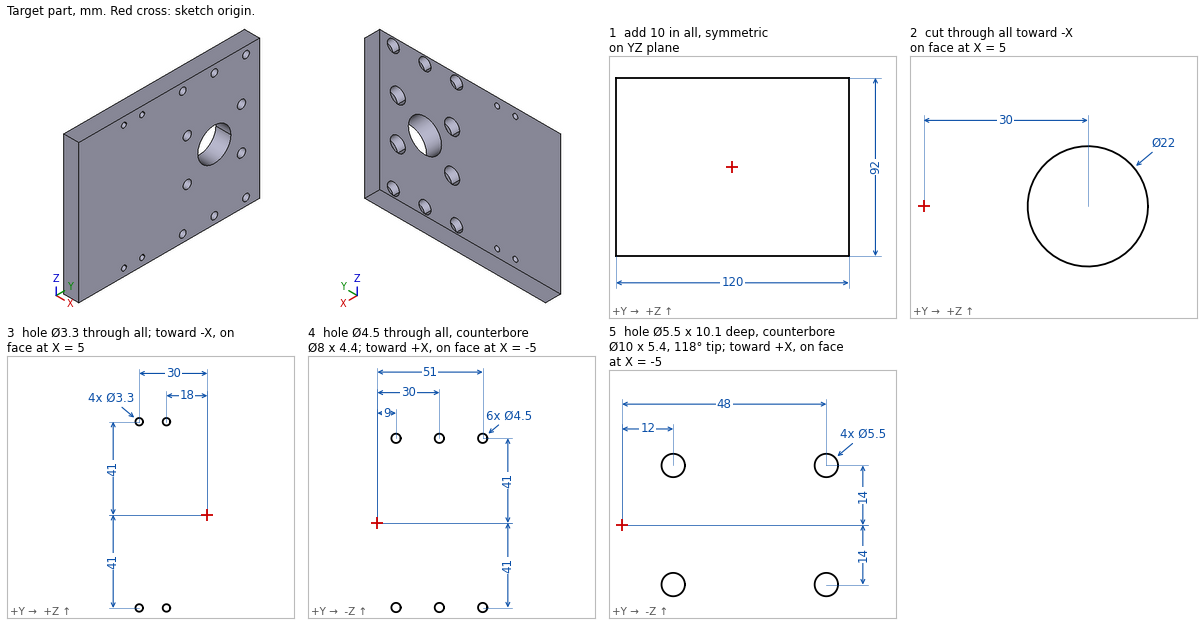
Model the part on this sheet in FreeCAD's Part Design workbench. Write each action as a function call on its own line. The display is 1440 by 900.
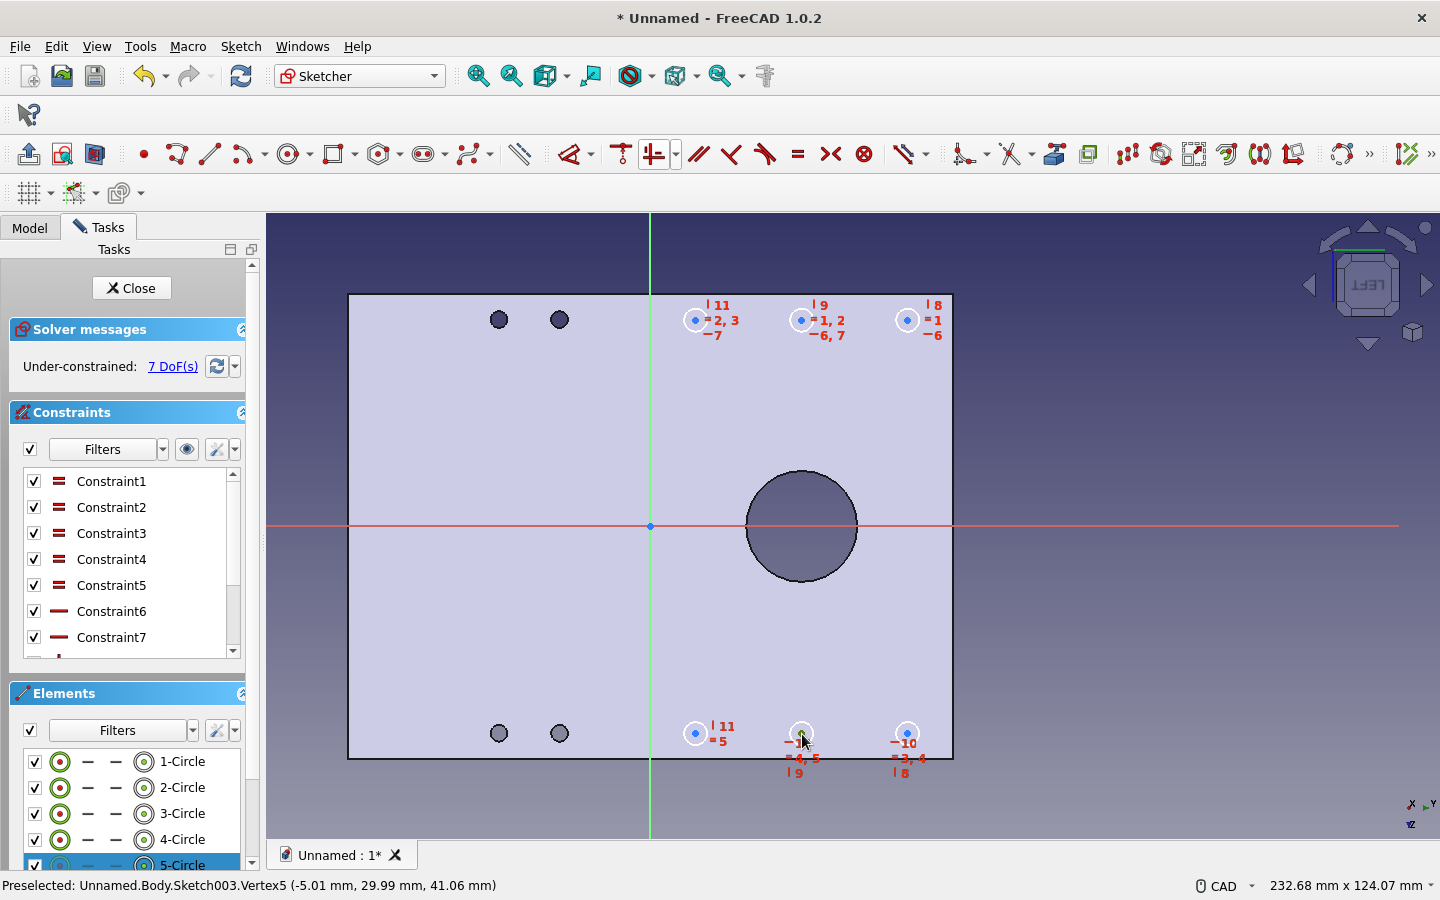
click(696, 734)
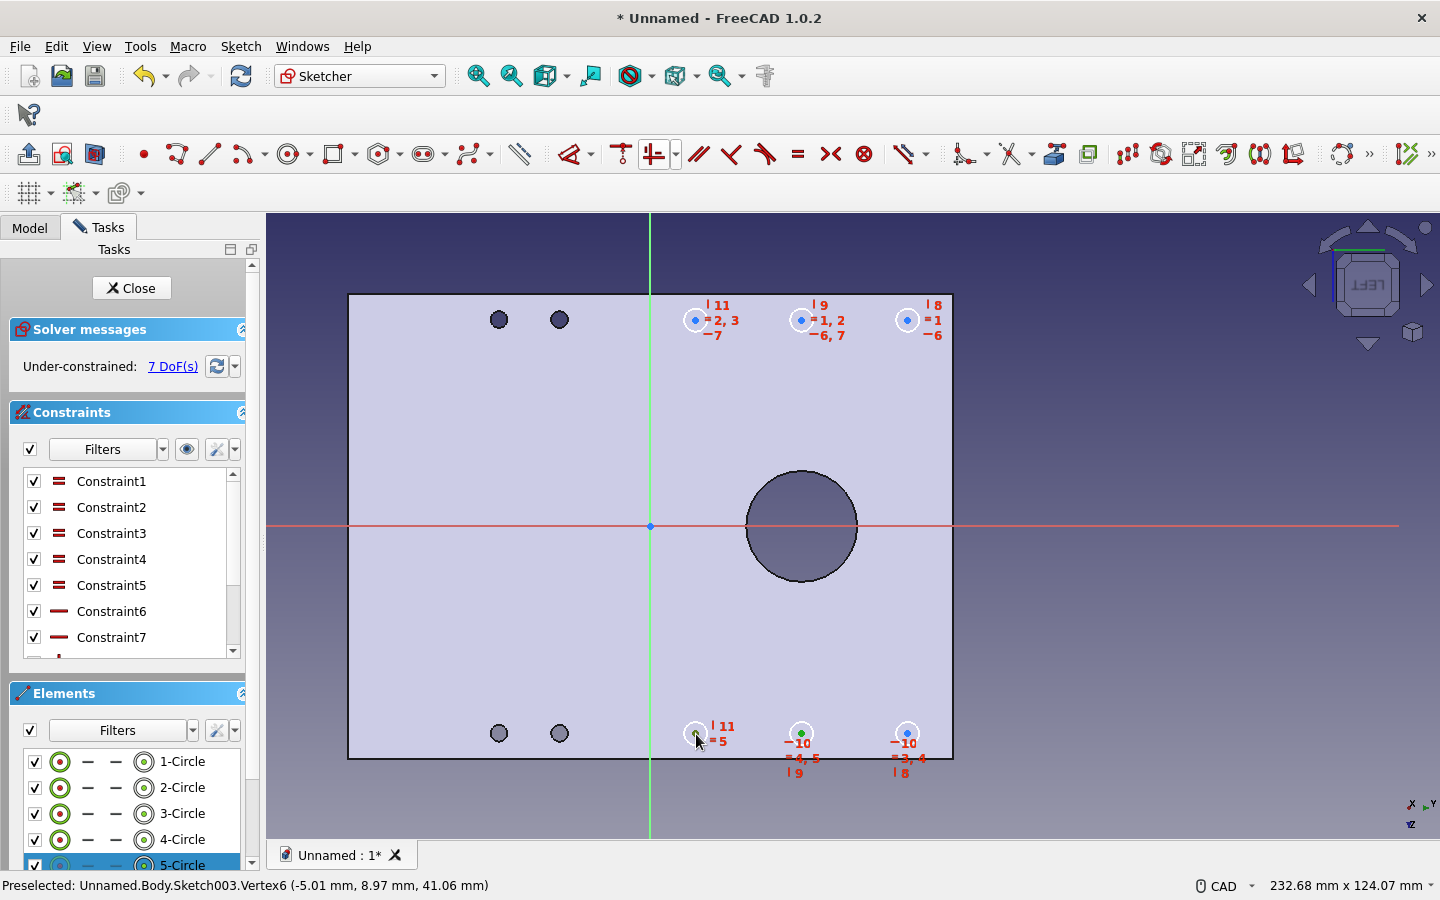
key(h)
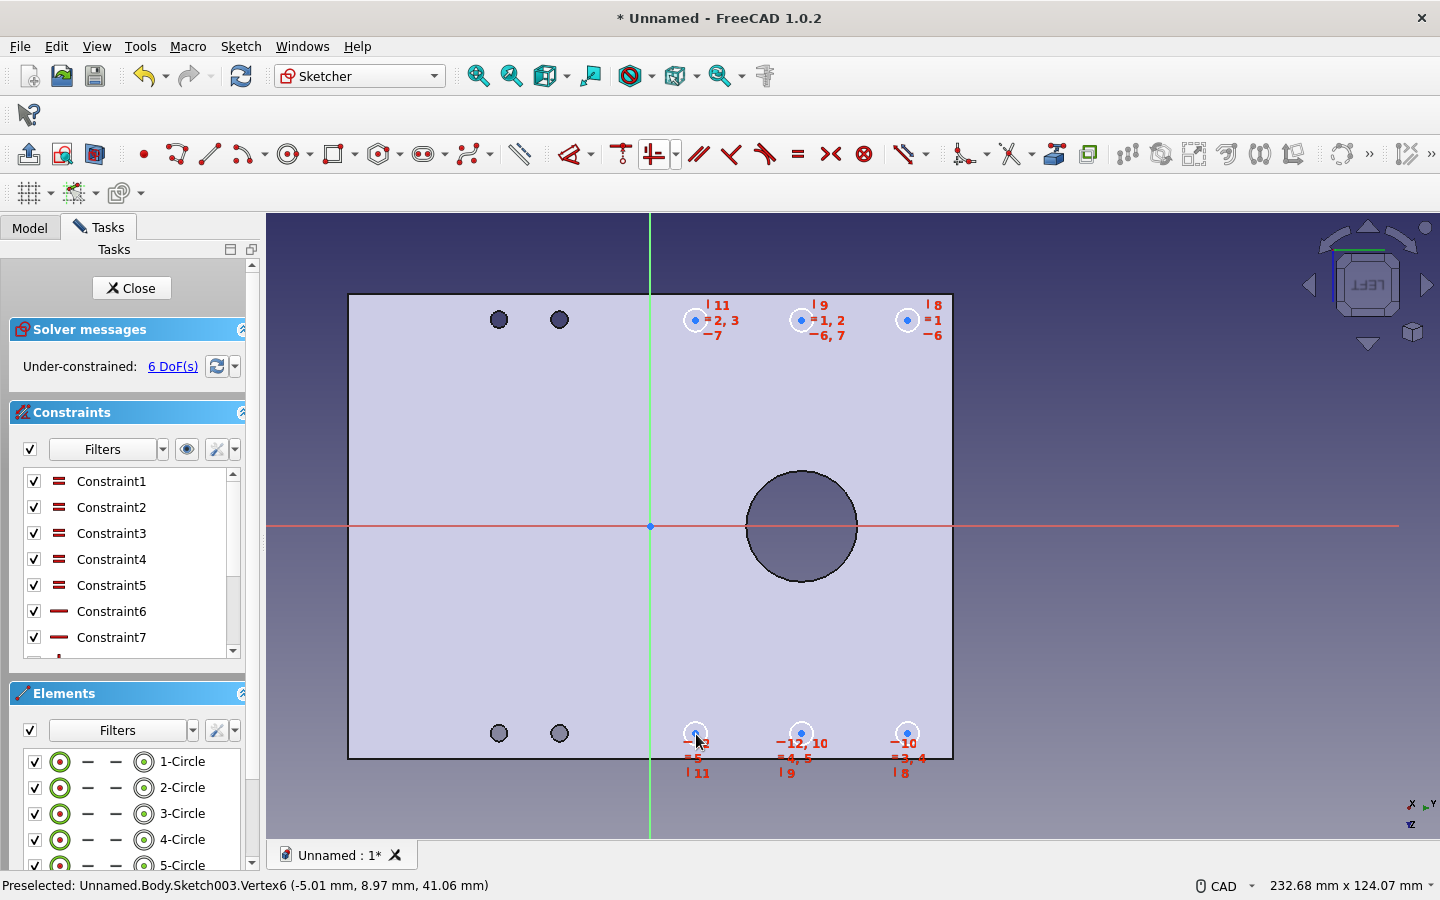
click(568, 154)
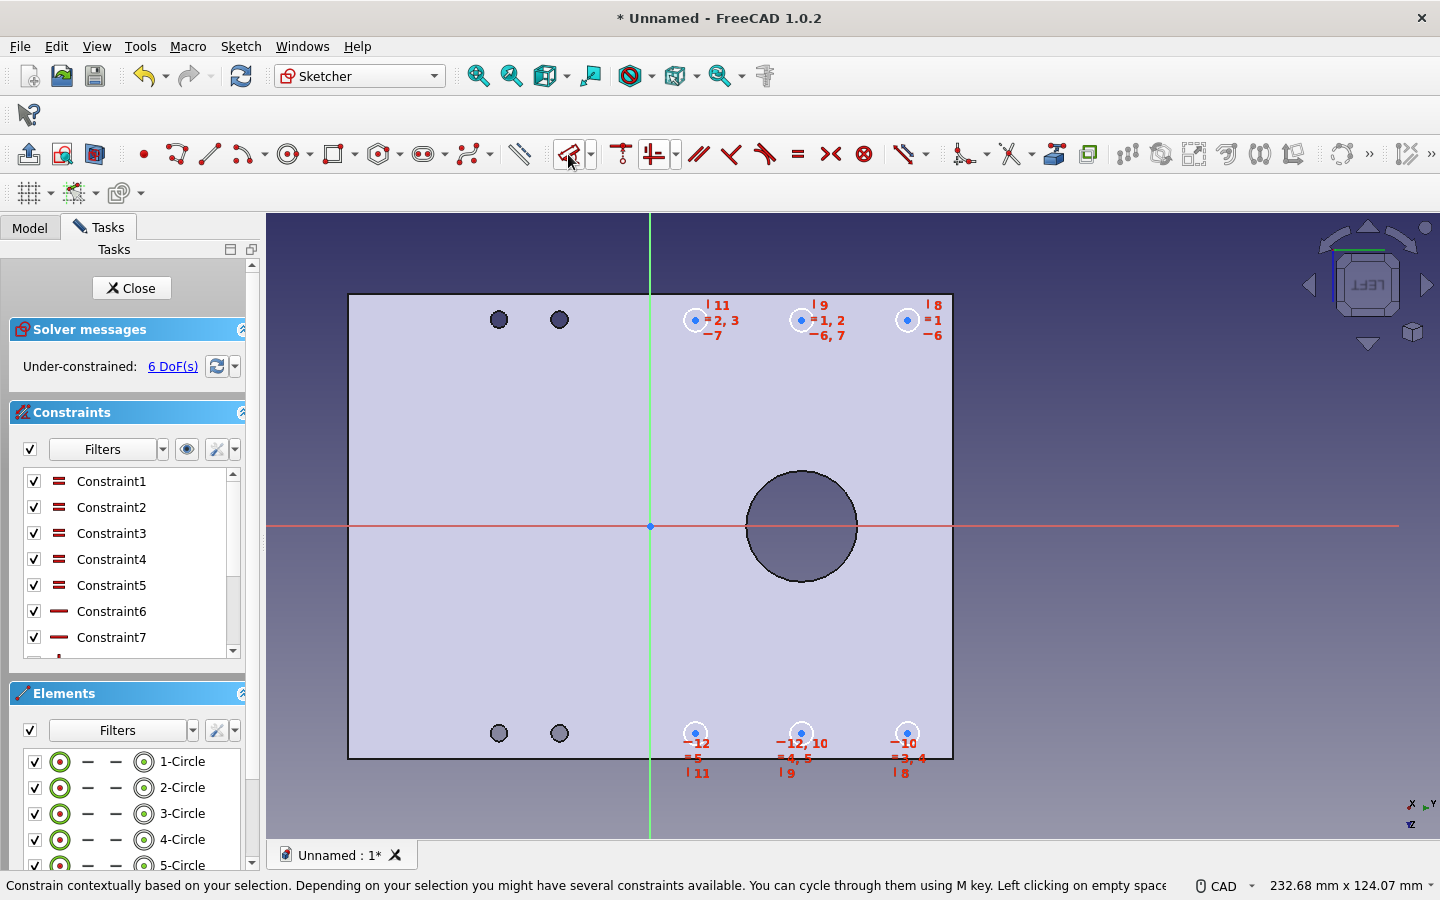
scroll(916, 312, up, 3)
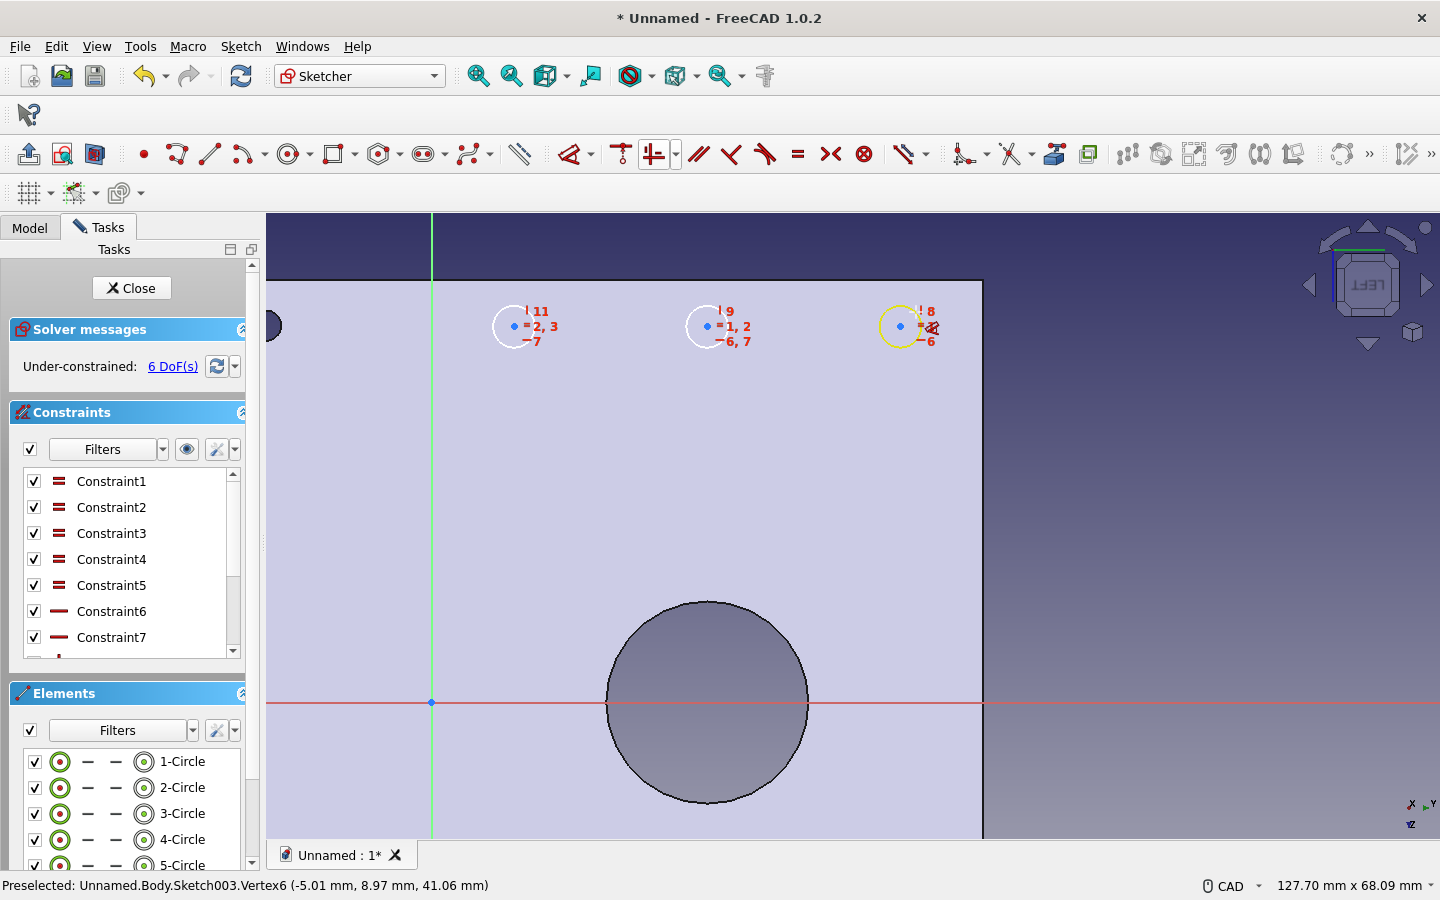
click(915, 312)
click(937, 289)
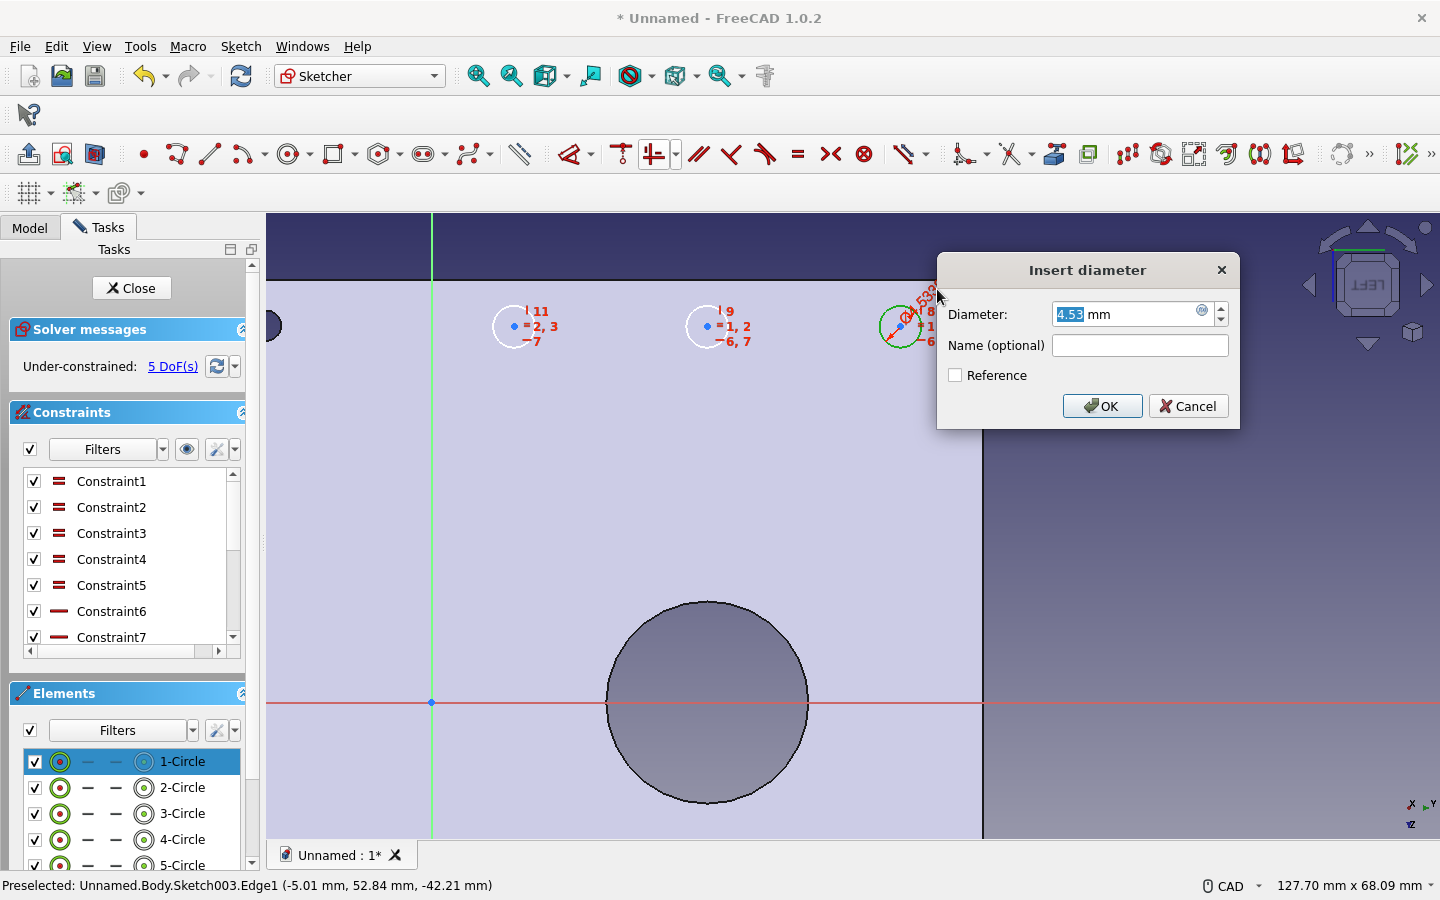
text(4.5)
key(Return)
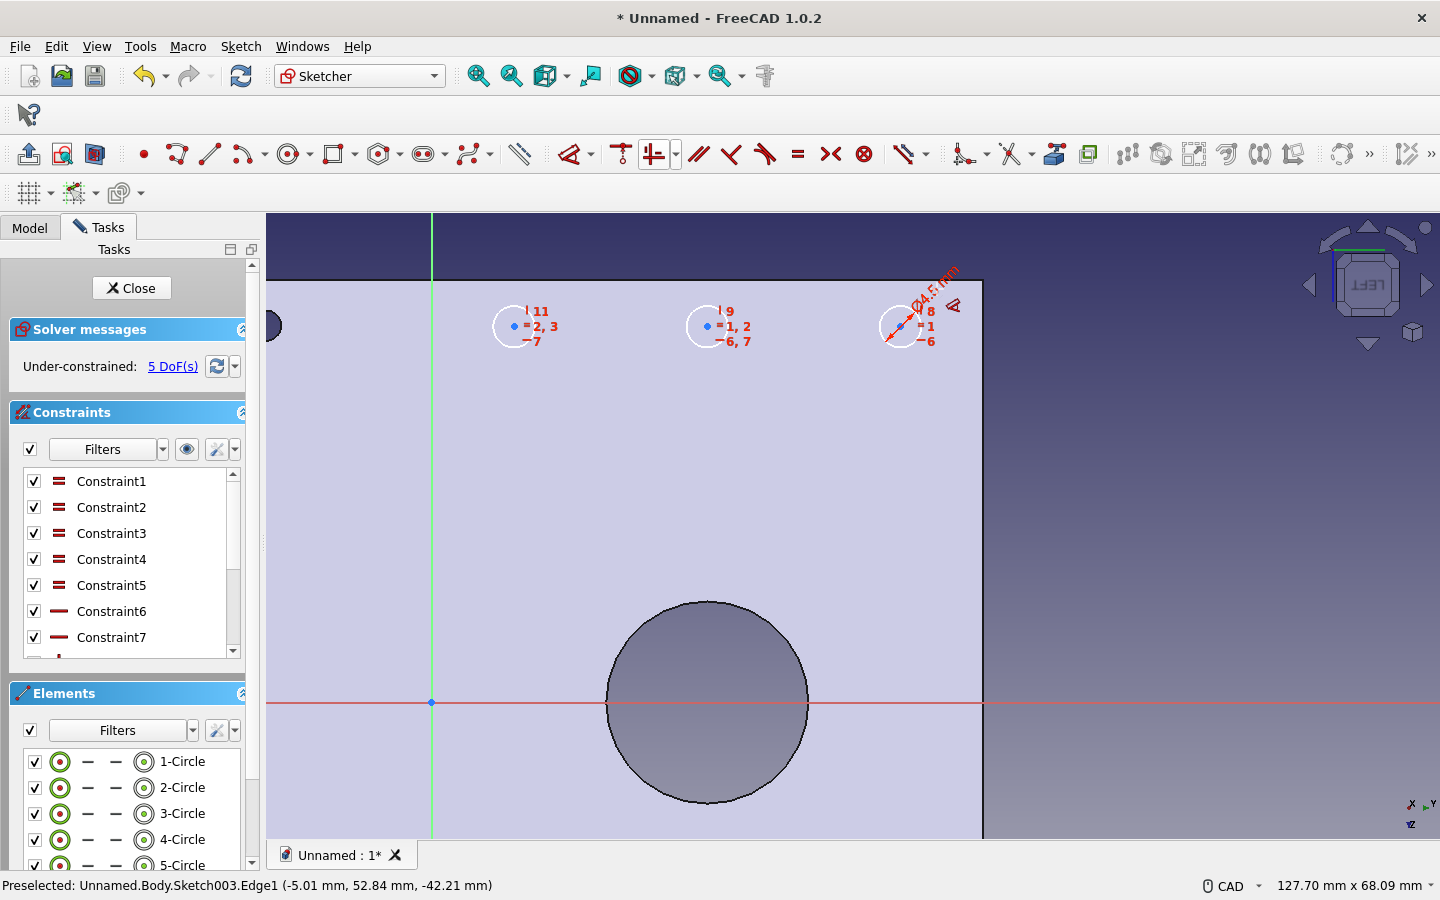
click(514, 327)
click(473, 293)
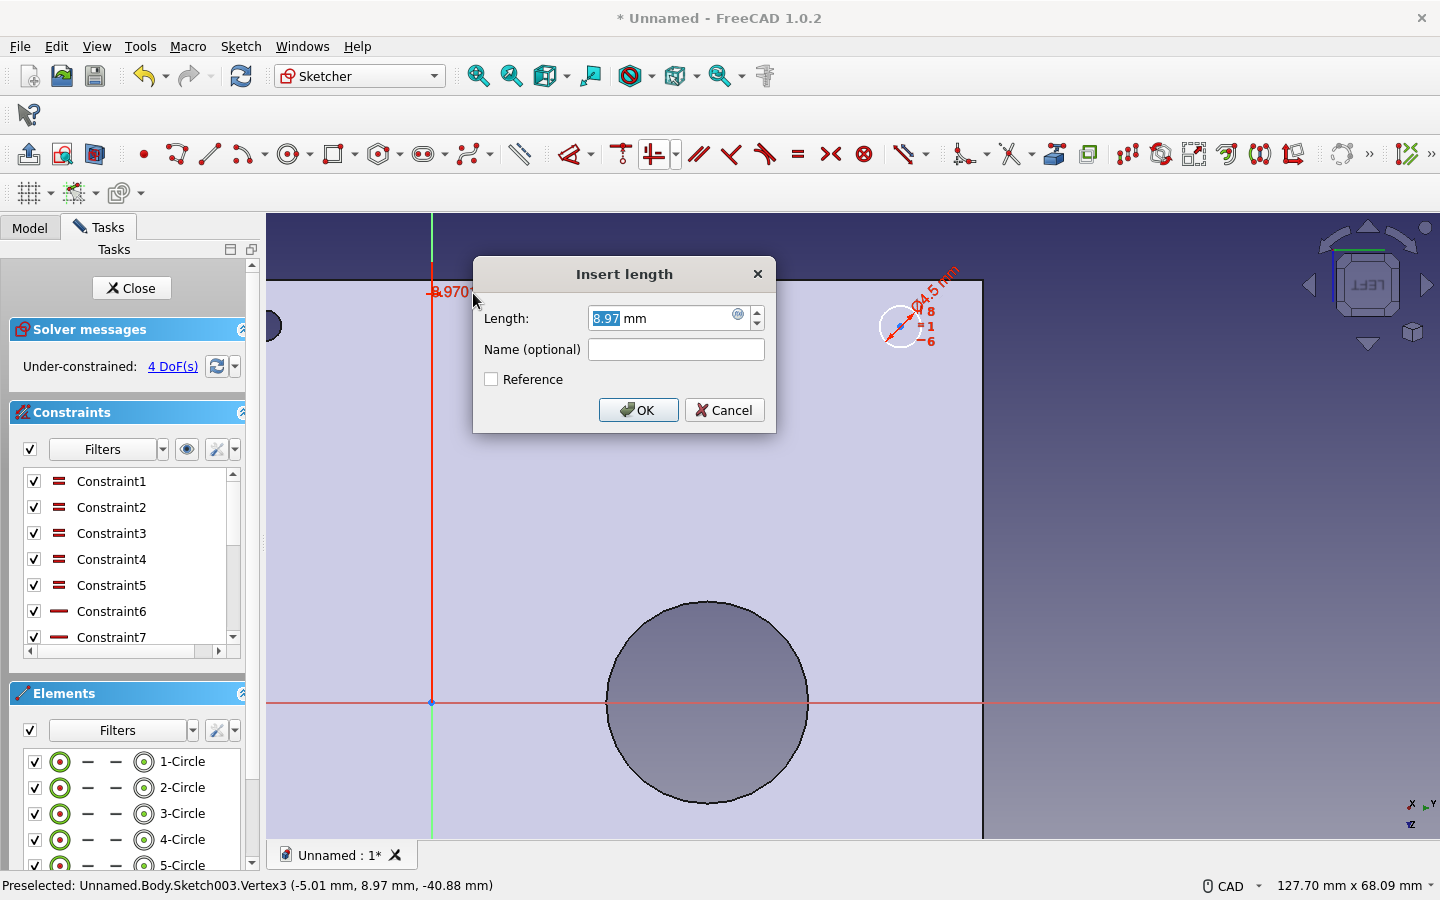
text(9)
key(Return)